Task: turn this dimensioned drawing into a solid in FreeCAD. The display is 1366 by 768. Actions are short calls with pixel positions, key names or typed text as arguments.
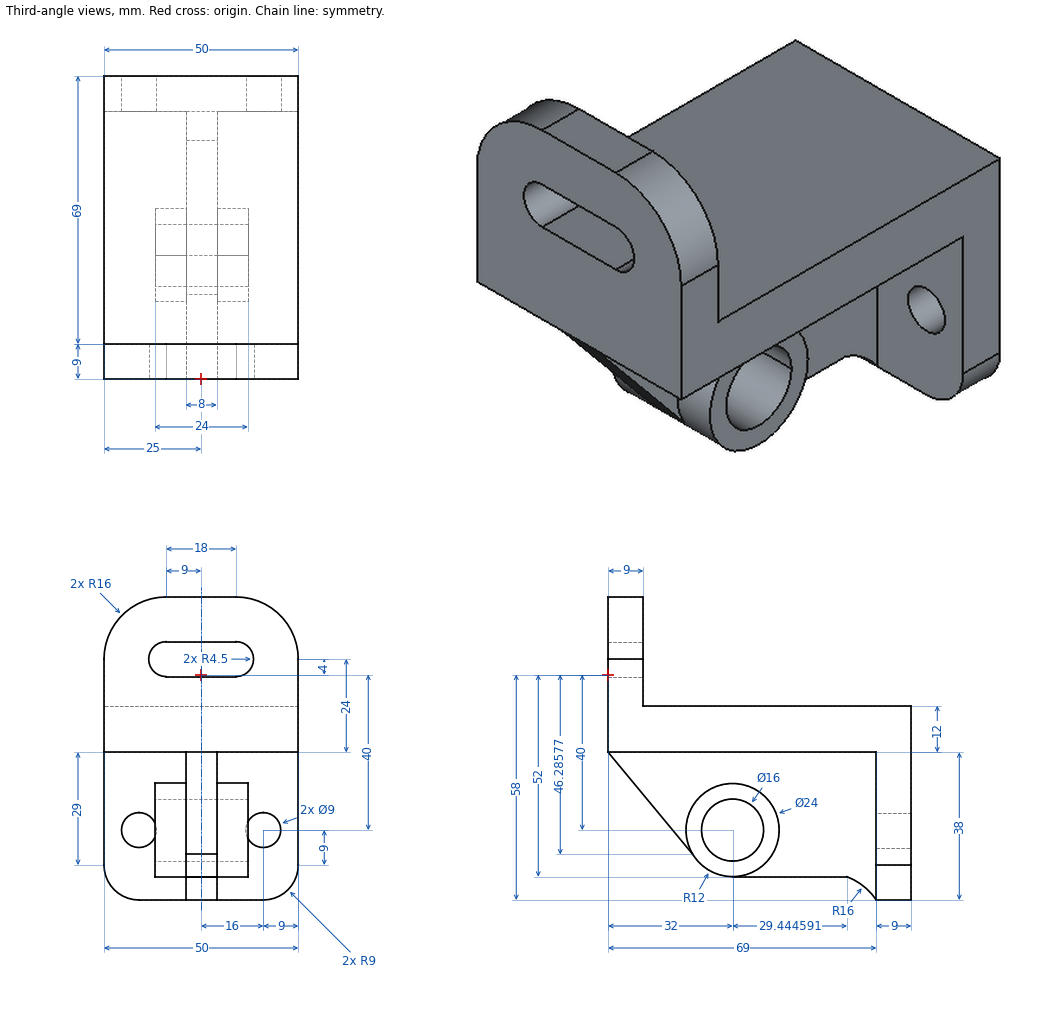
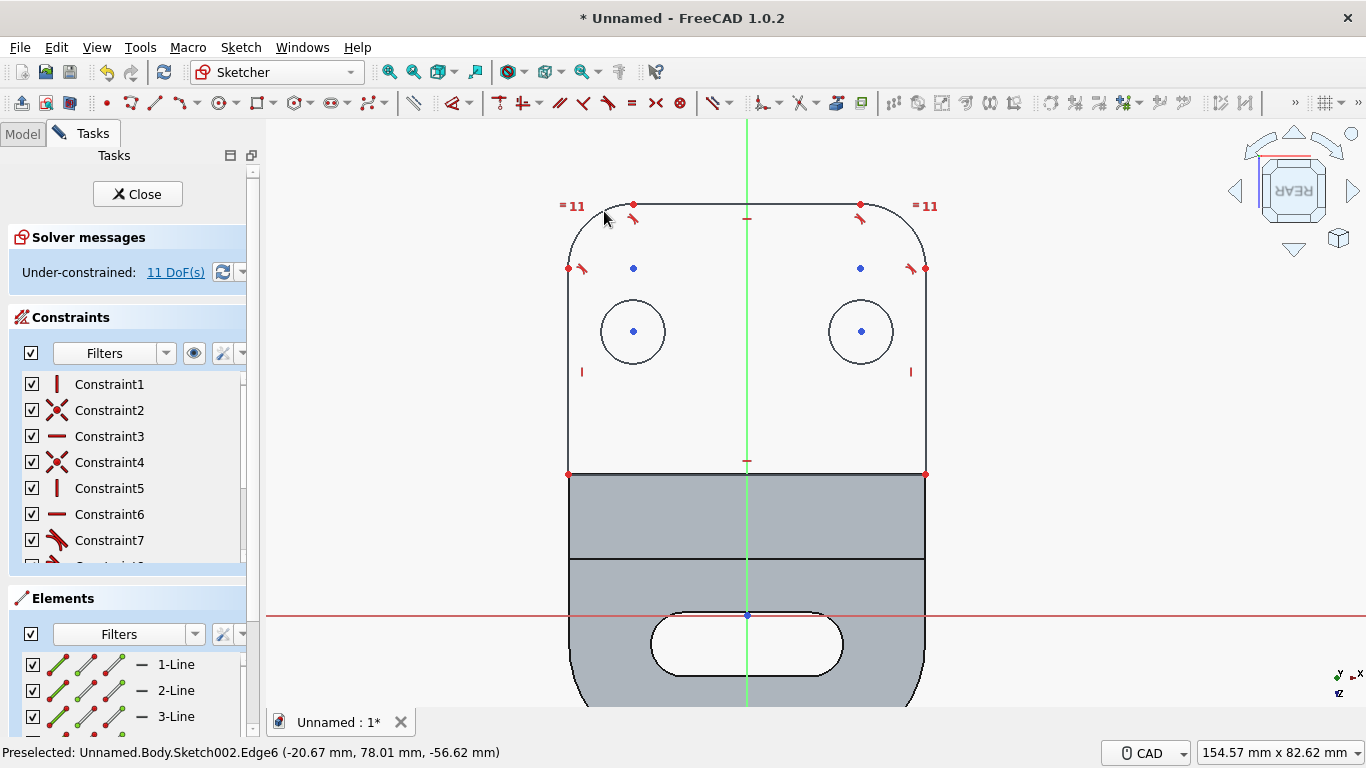
click(883, 309)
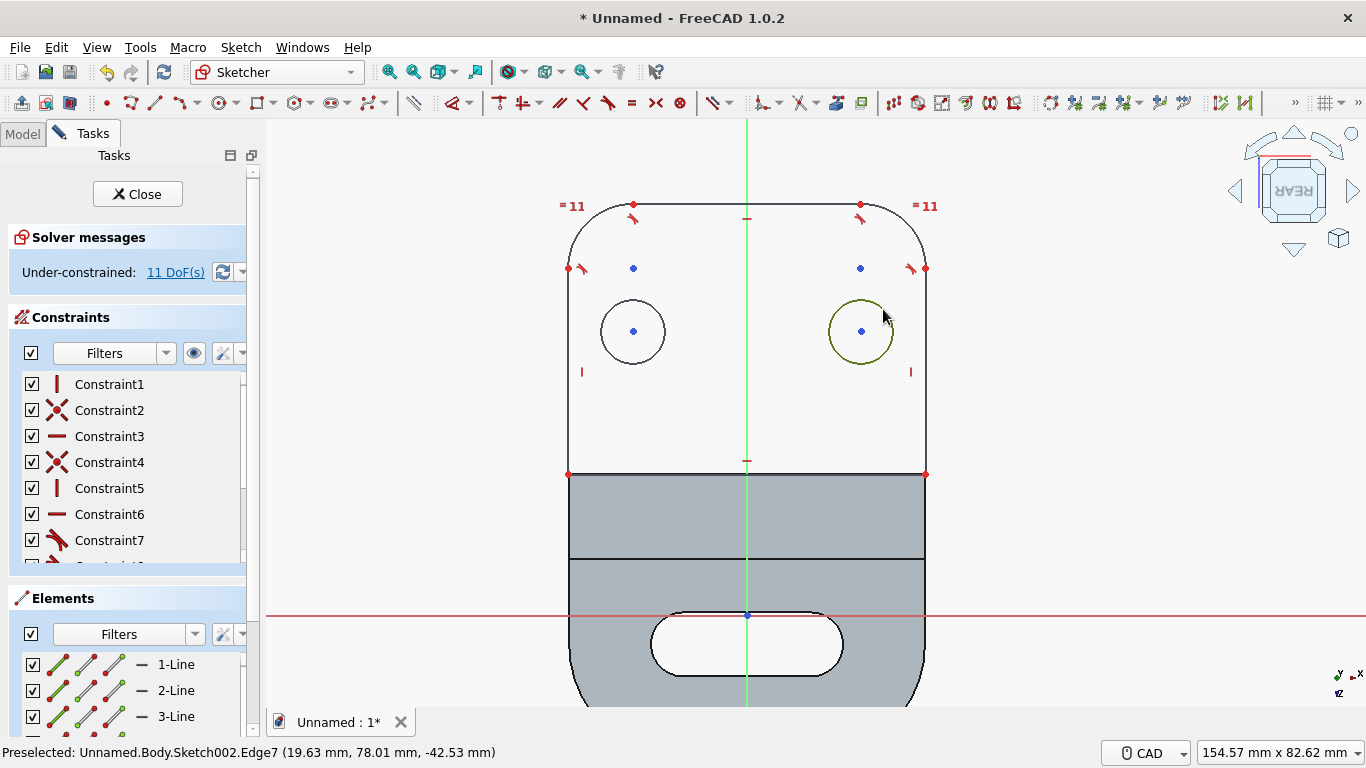
click(655, 309)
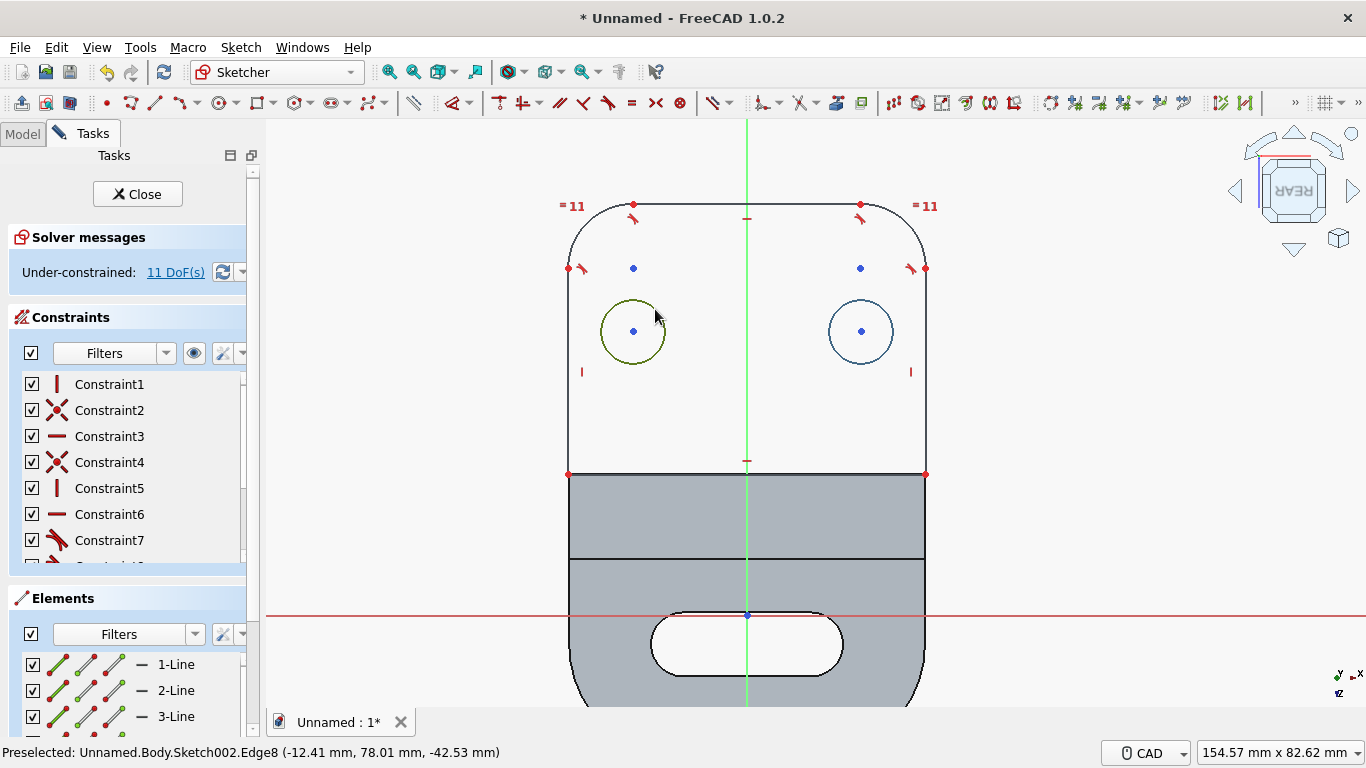
click(632, 104)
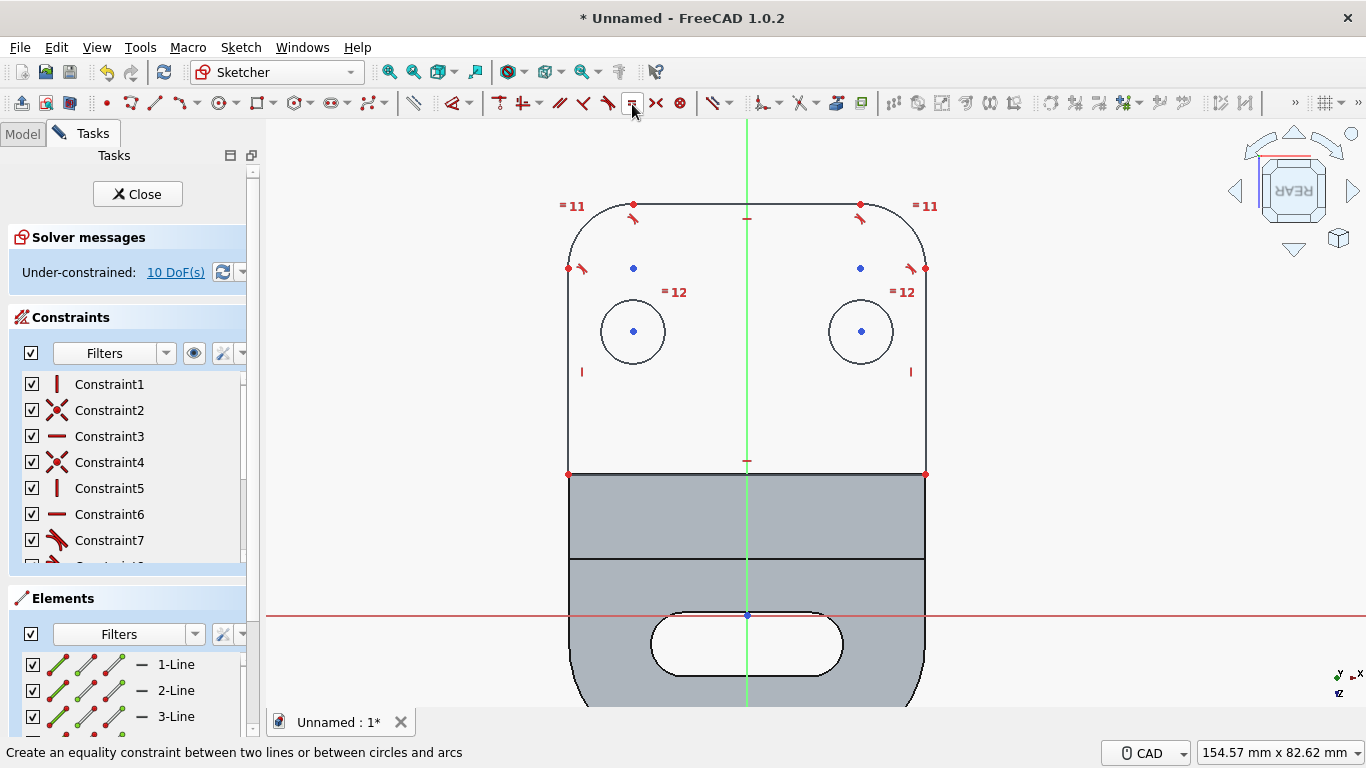
click(861, 332)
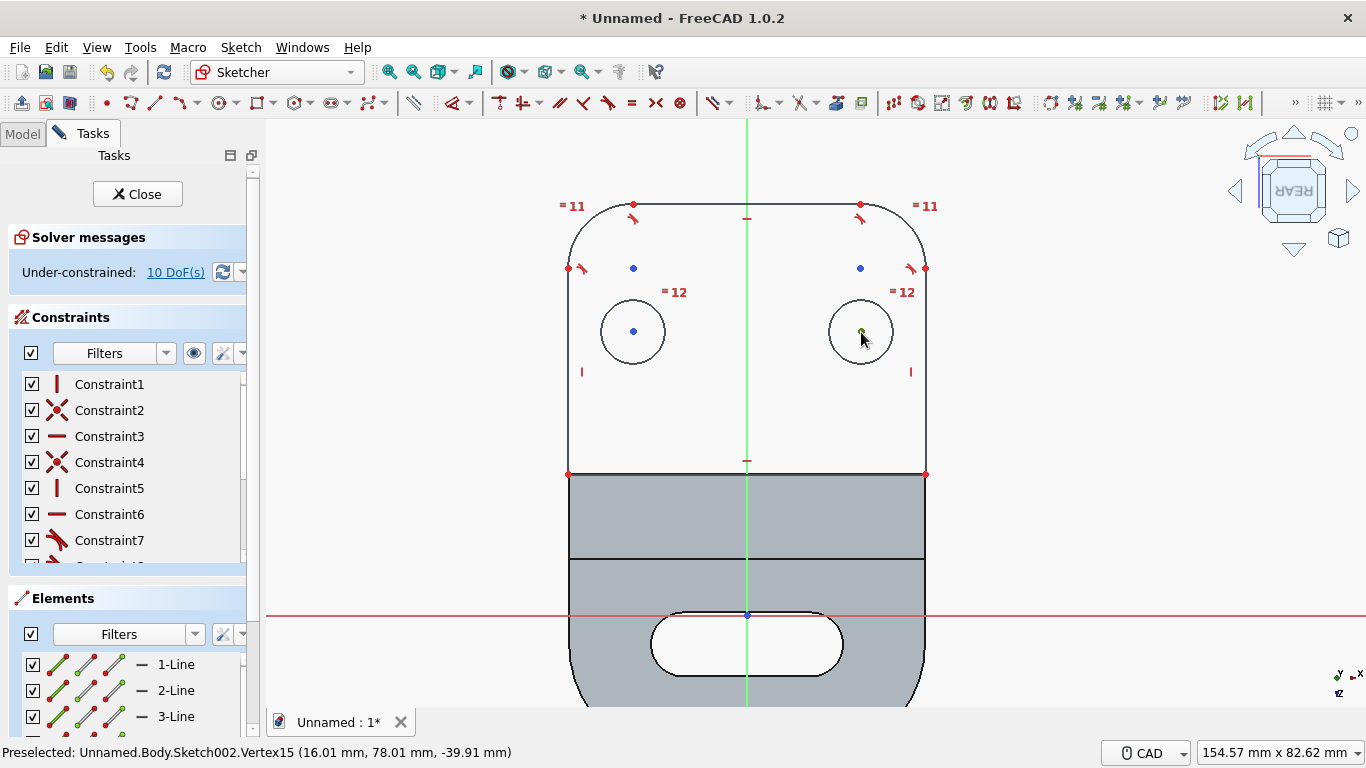
click(633, 332)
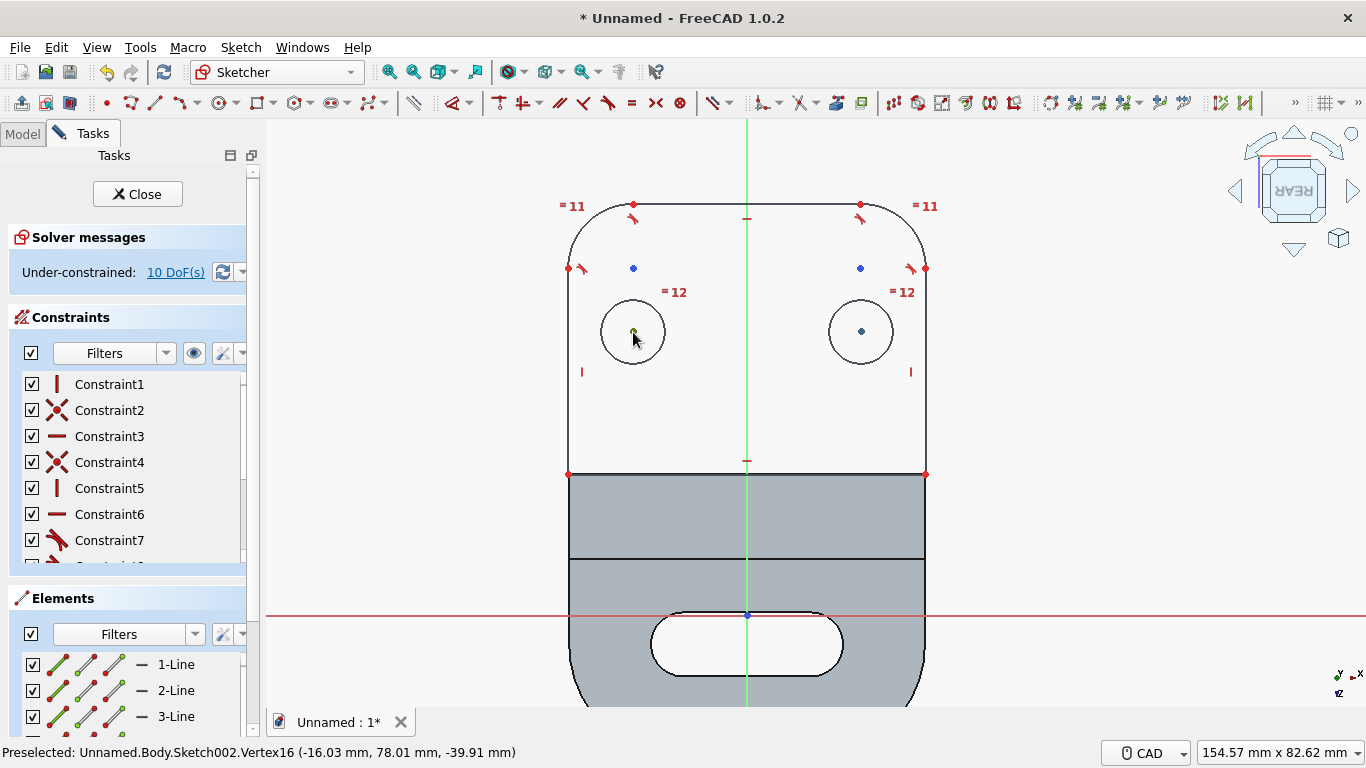
click(747, 565)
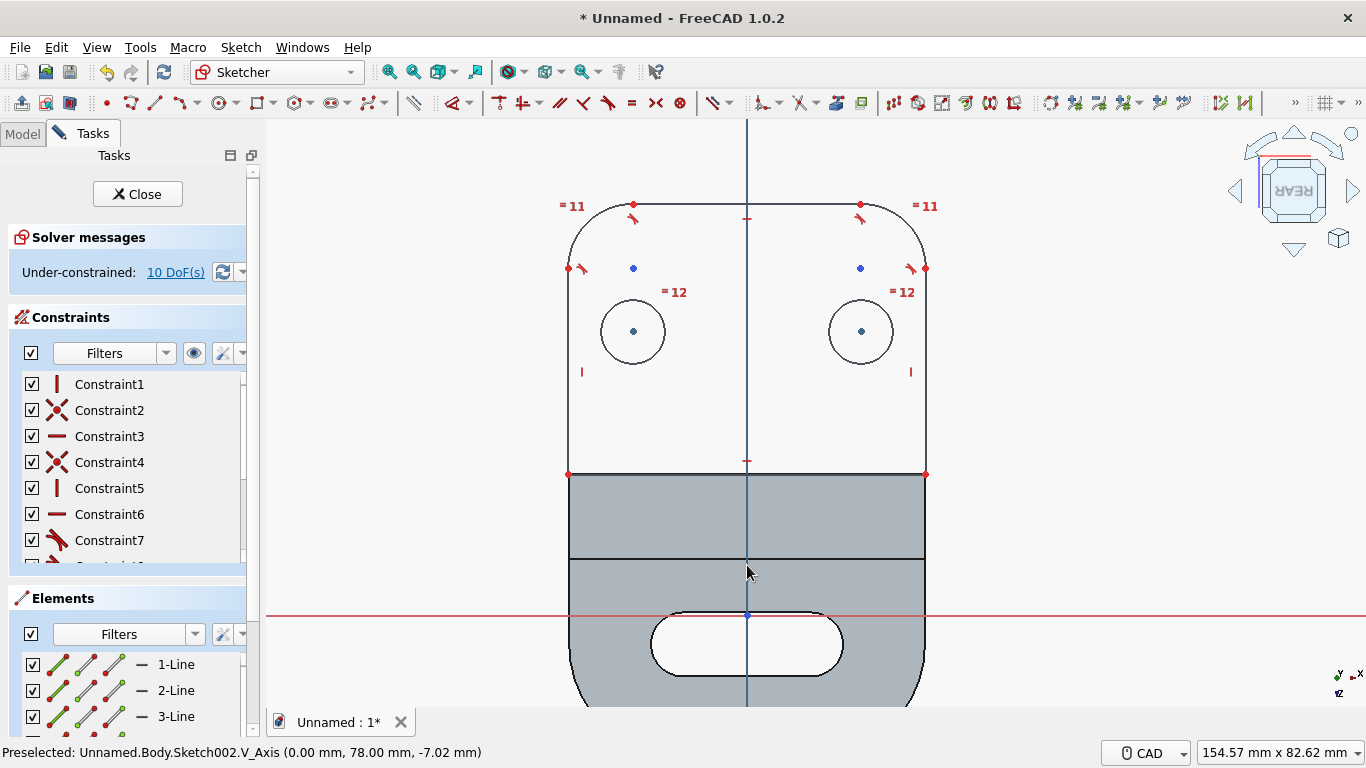
click(656, 104)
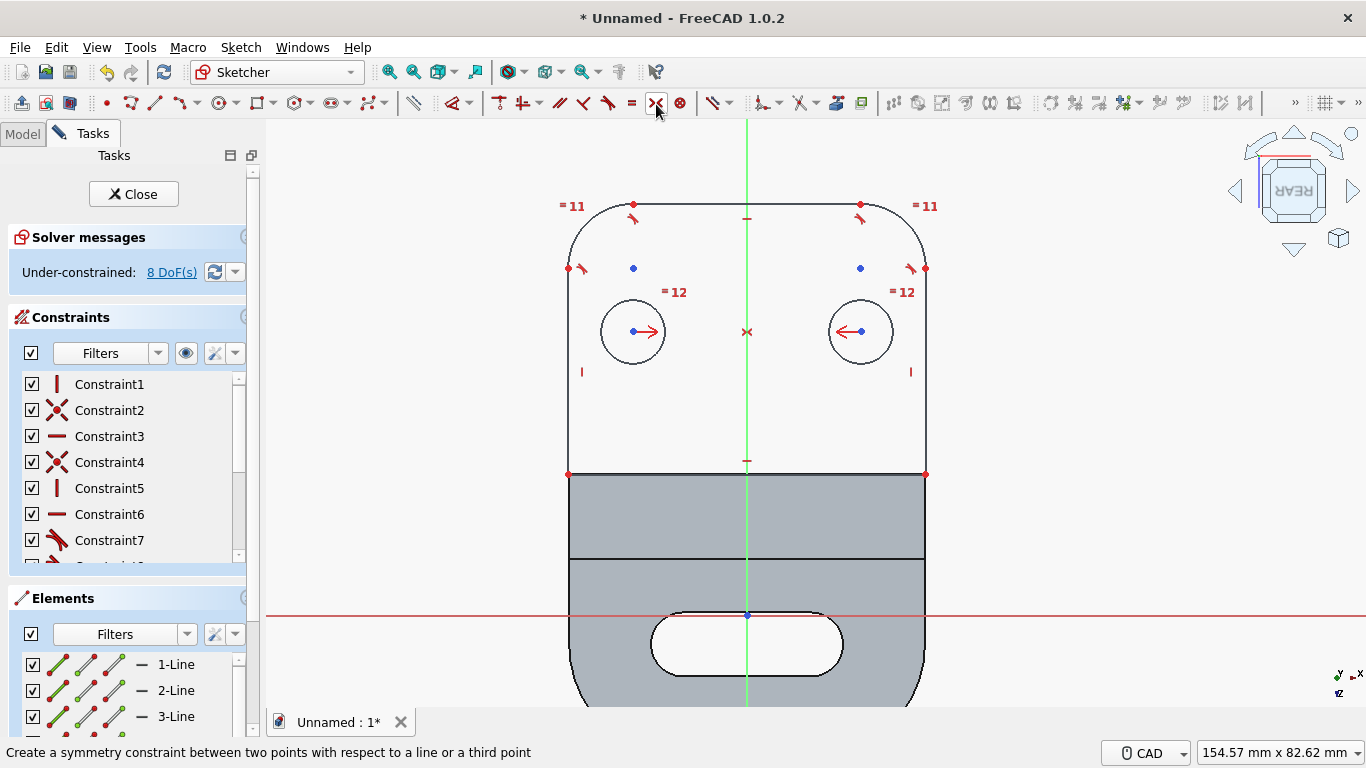
click(452, 104)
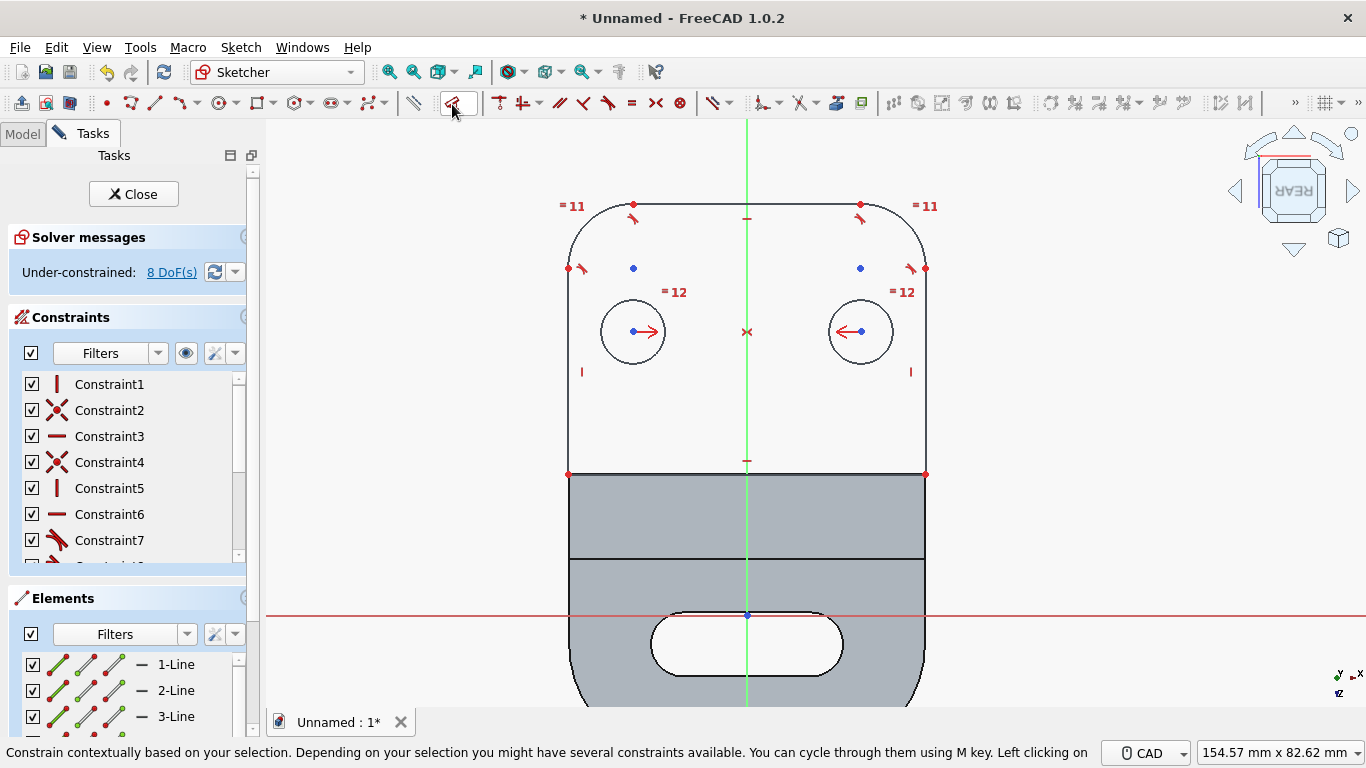
click(919, 239)
click(947, 224)